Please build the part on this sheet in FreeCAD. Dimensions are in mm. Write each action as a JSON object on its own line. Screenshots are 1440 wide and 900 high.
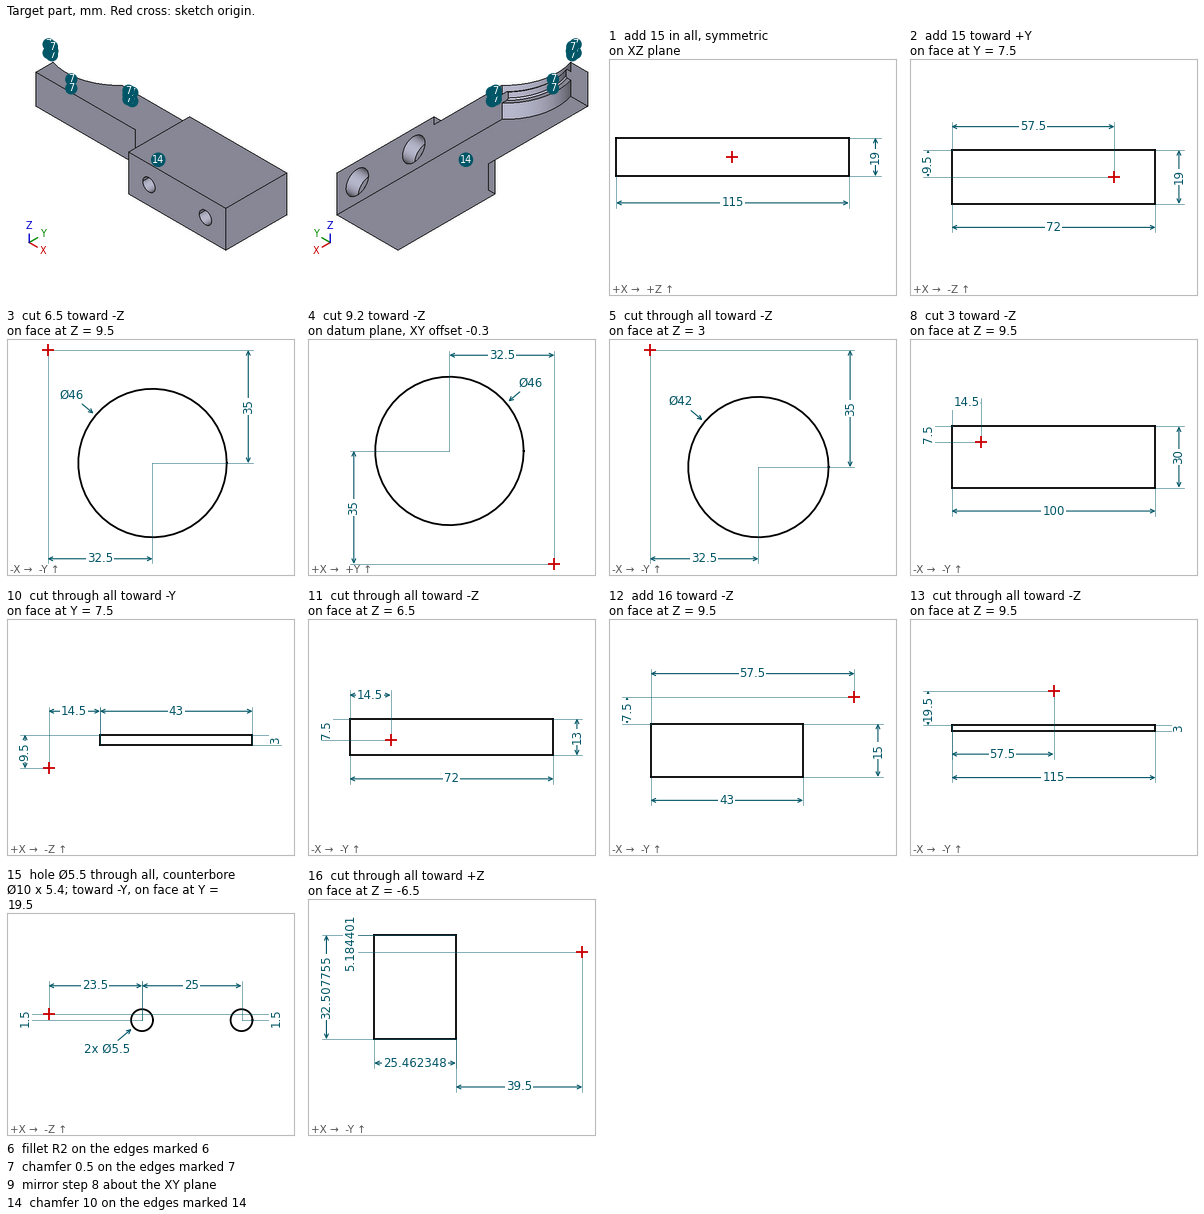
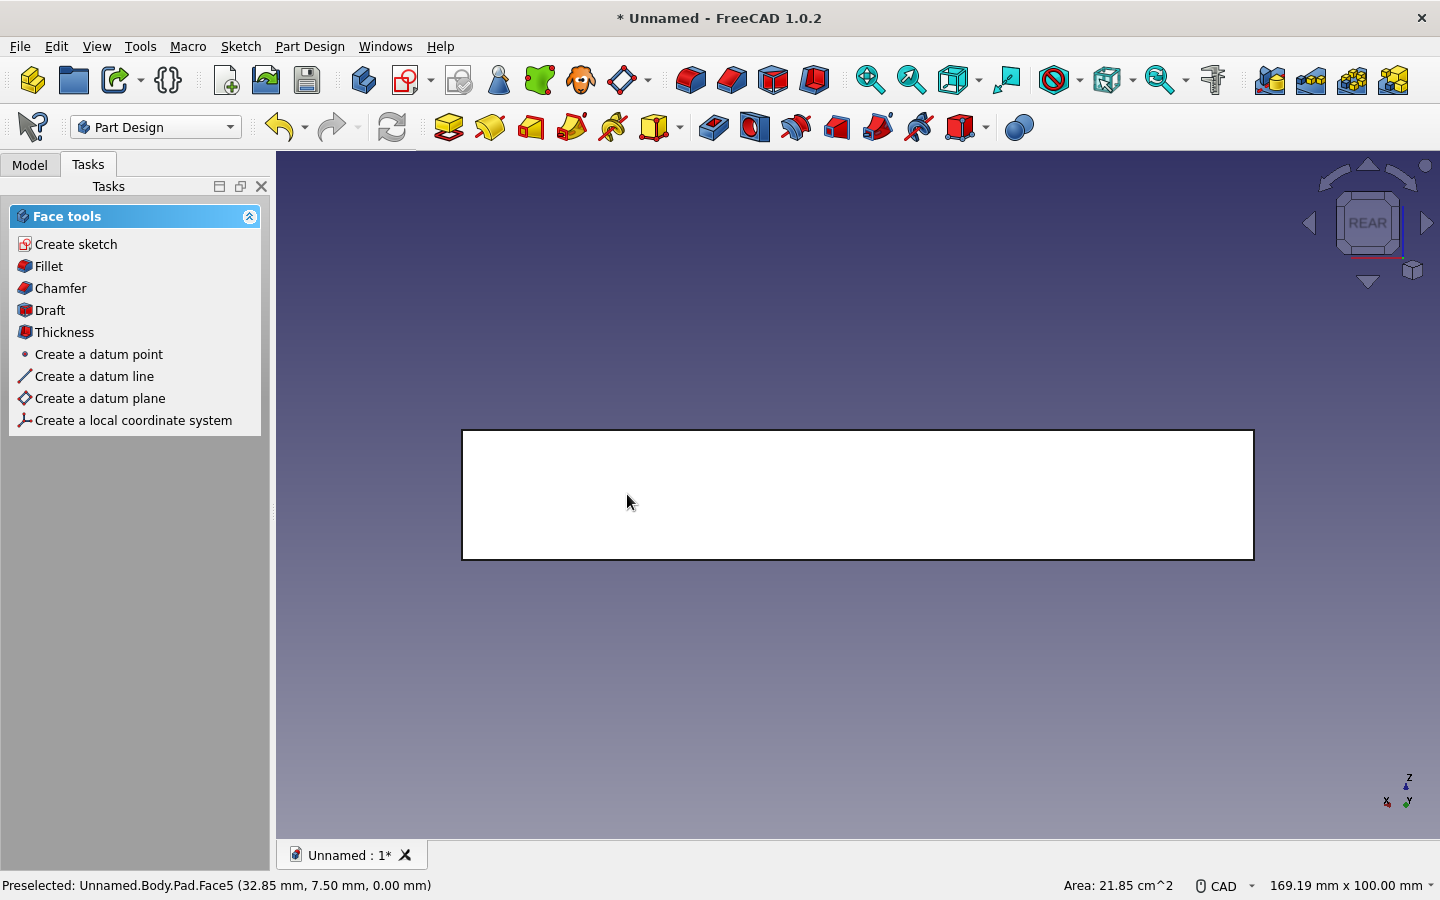
{"action": "left_click", "coordinate": [404, 80]}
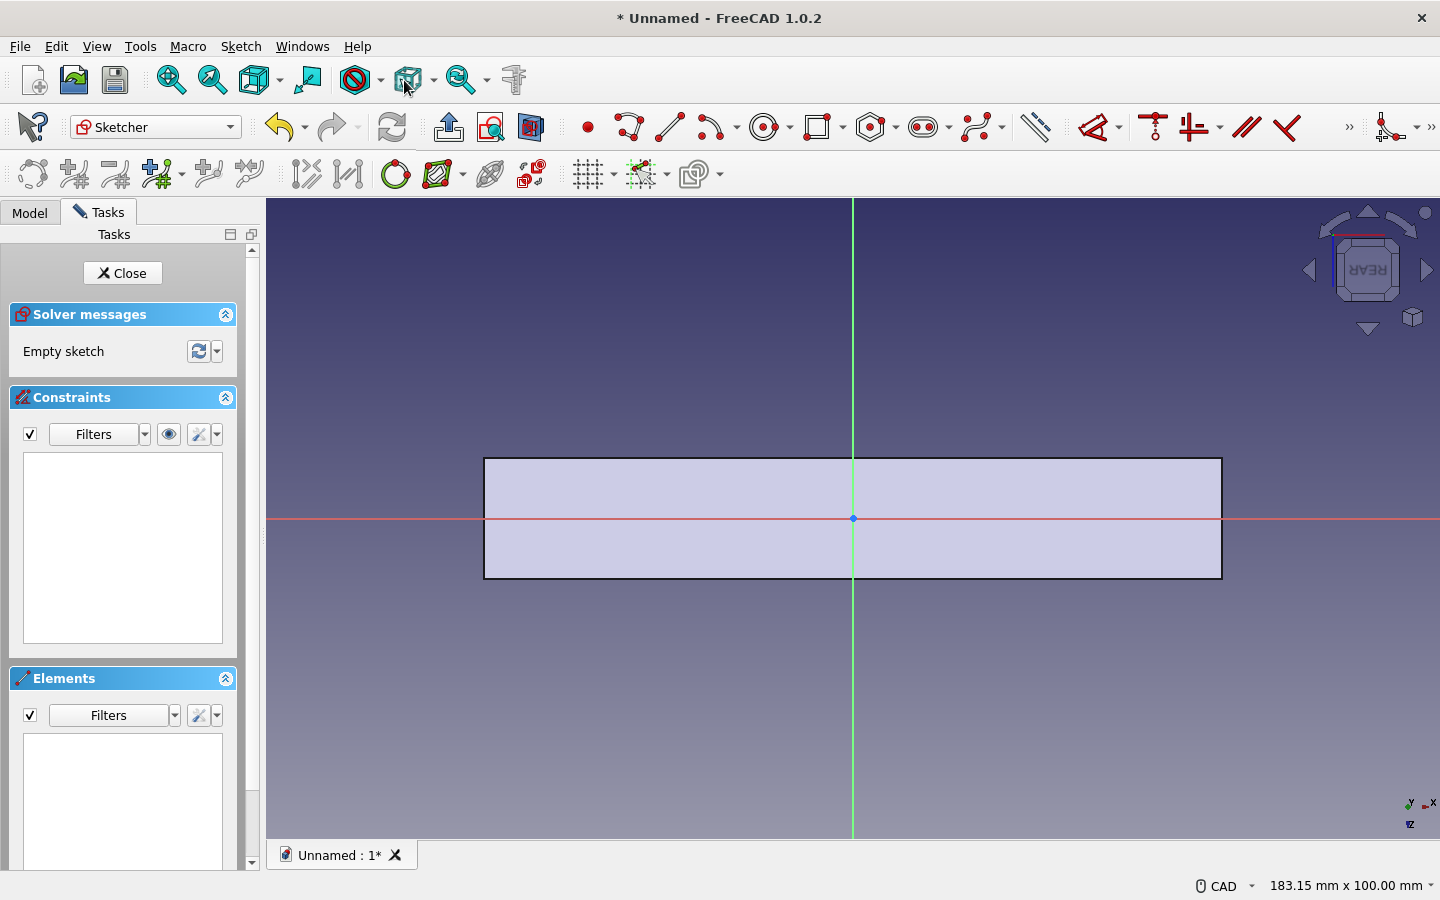
{"action": "scroll", "coordinate": [574, 519], "scroll_direction": "up", "scroll_amount": 2}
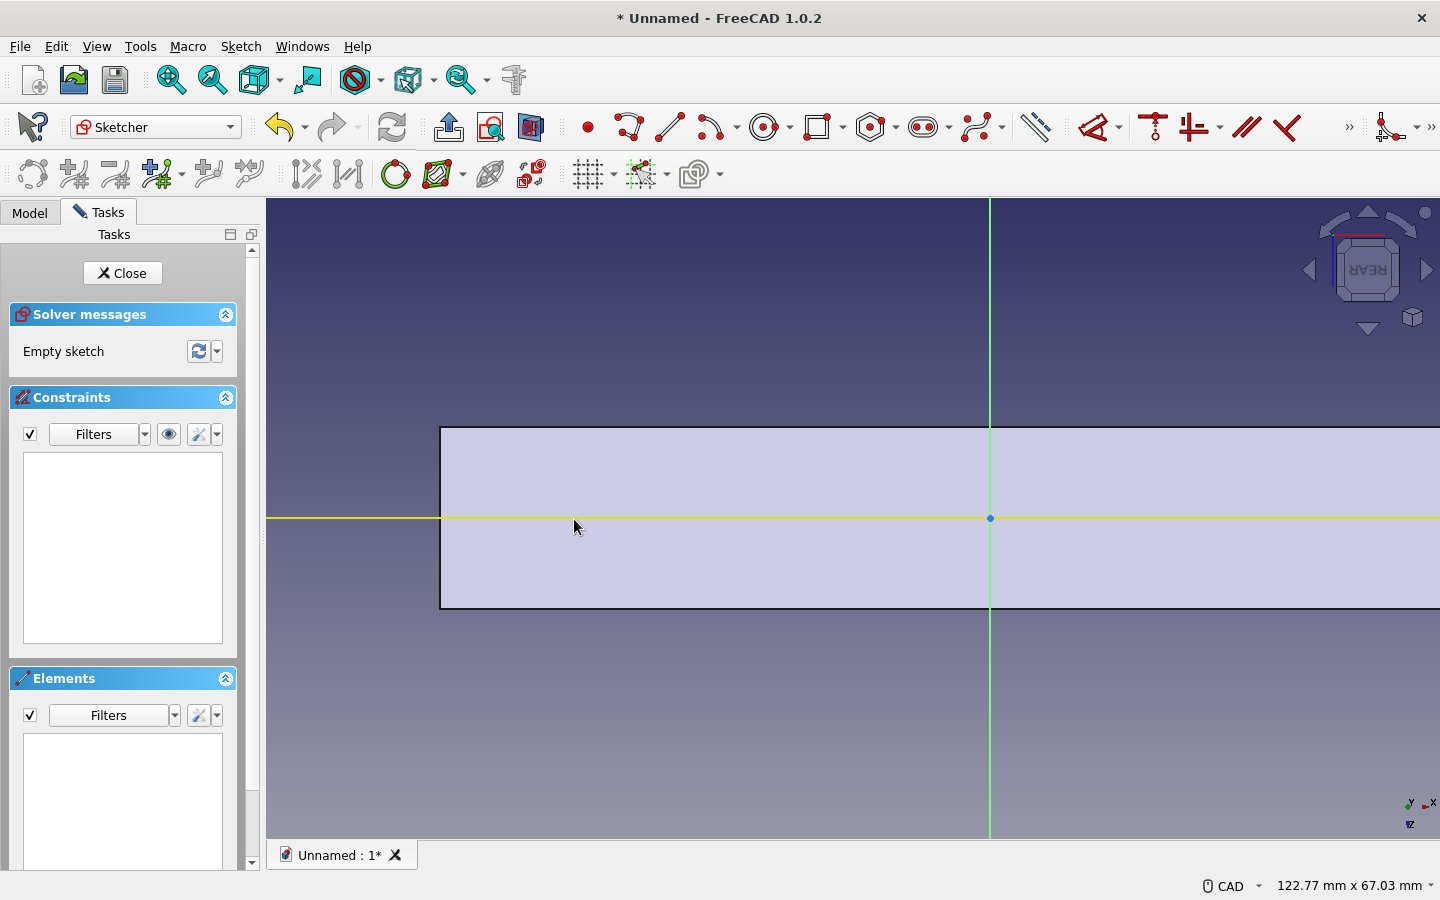
{"action": "left_click", "coordinate": [816, 128]}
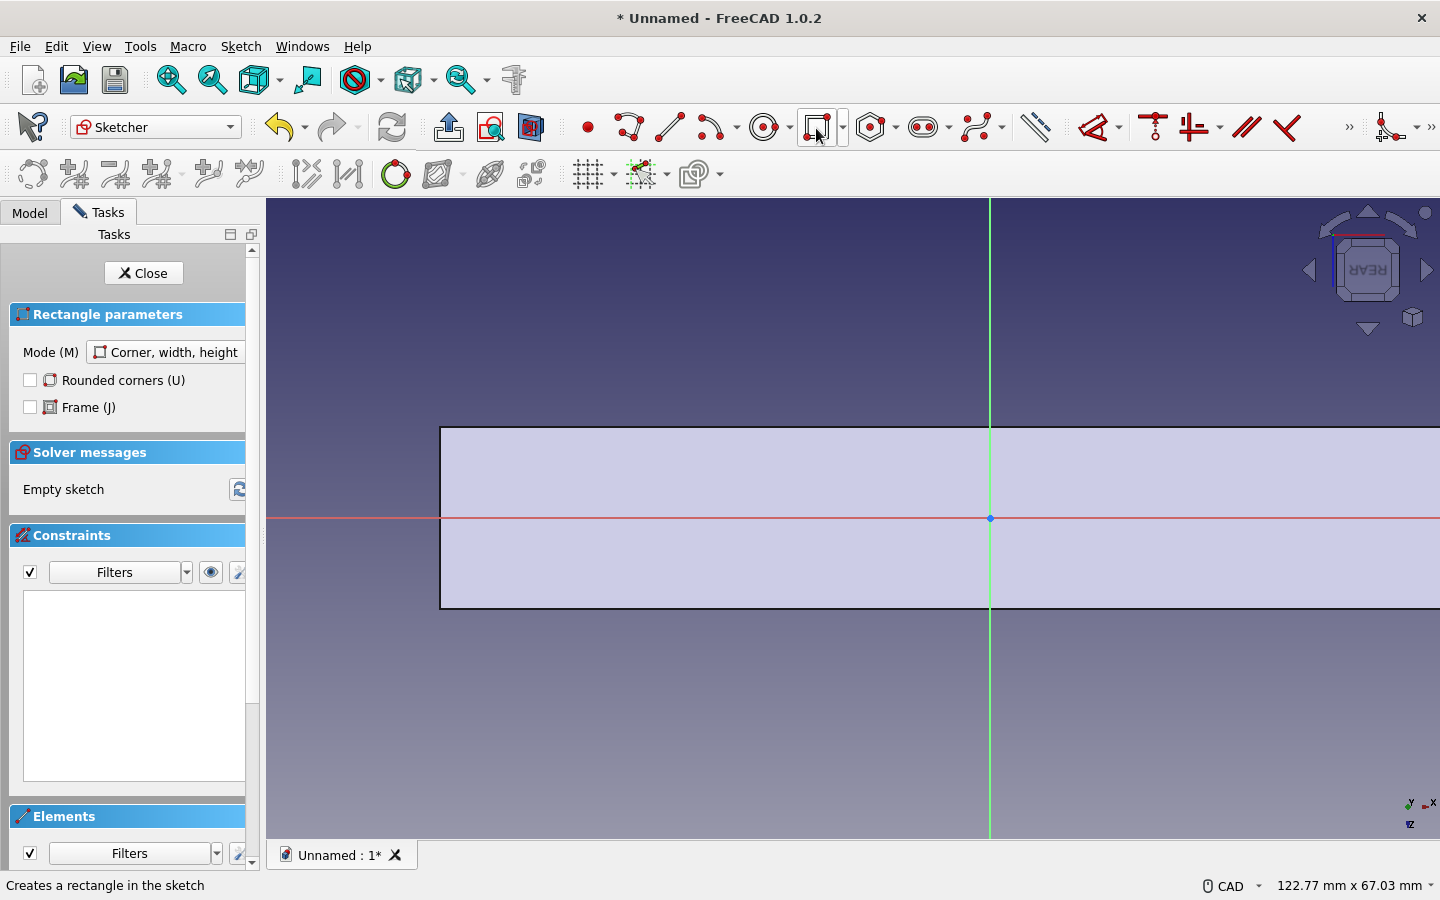
{"action": "left_click", "coordinate": [440, 427]}
{"action": "mouse_move", "coordinate": [1129, 609]}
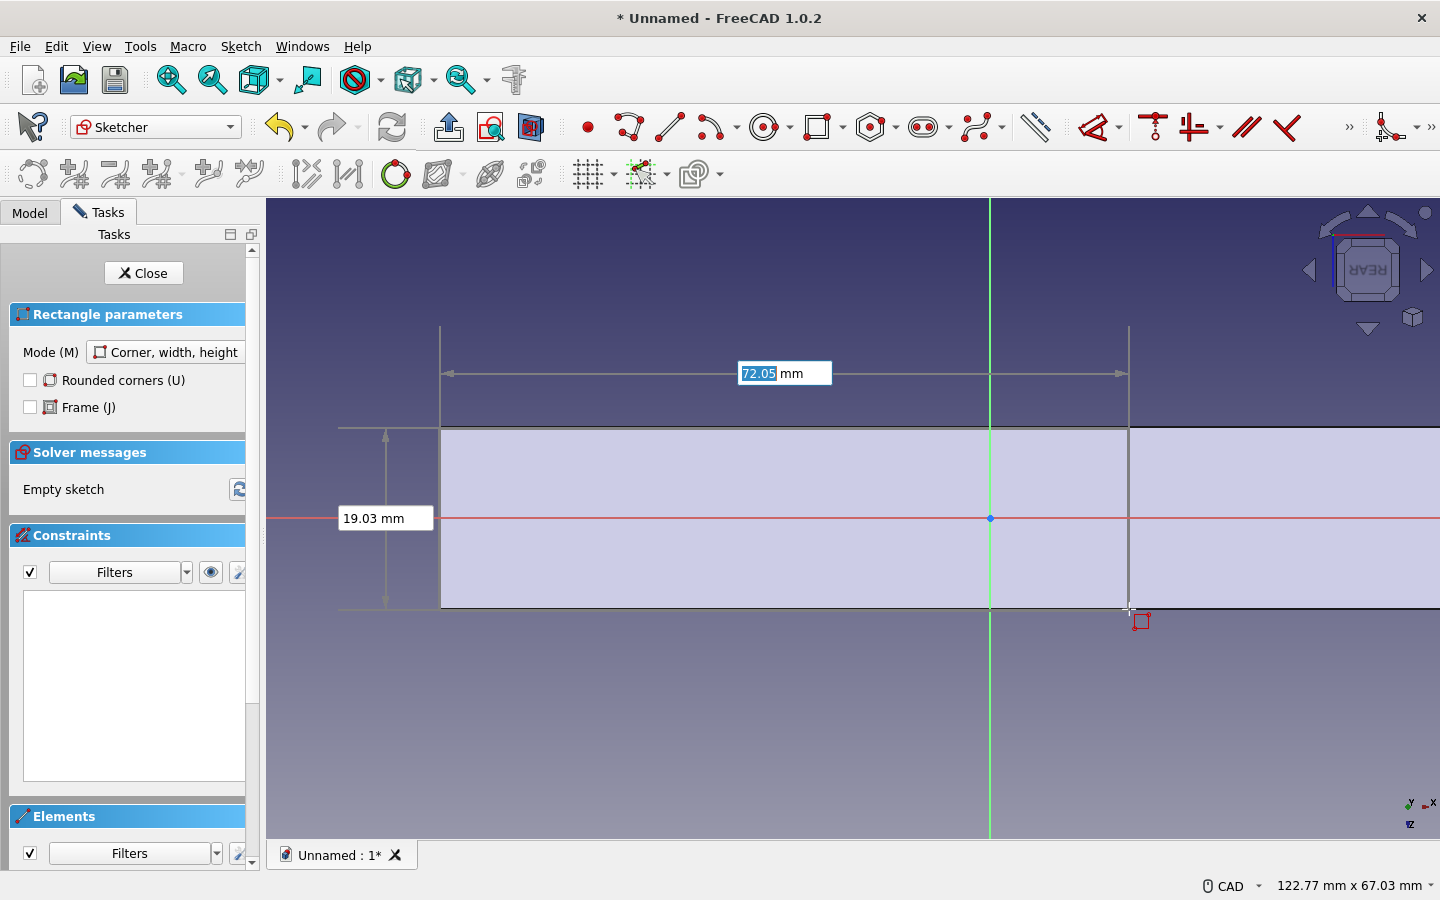
{"action": "type", "text": "72"}
{"action": "key", "text": "Tab"}
{"action": "type", "text": "19"}
{"action": "key", "text": "Return"}
{"action": "key", "text": "Escape"}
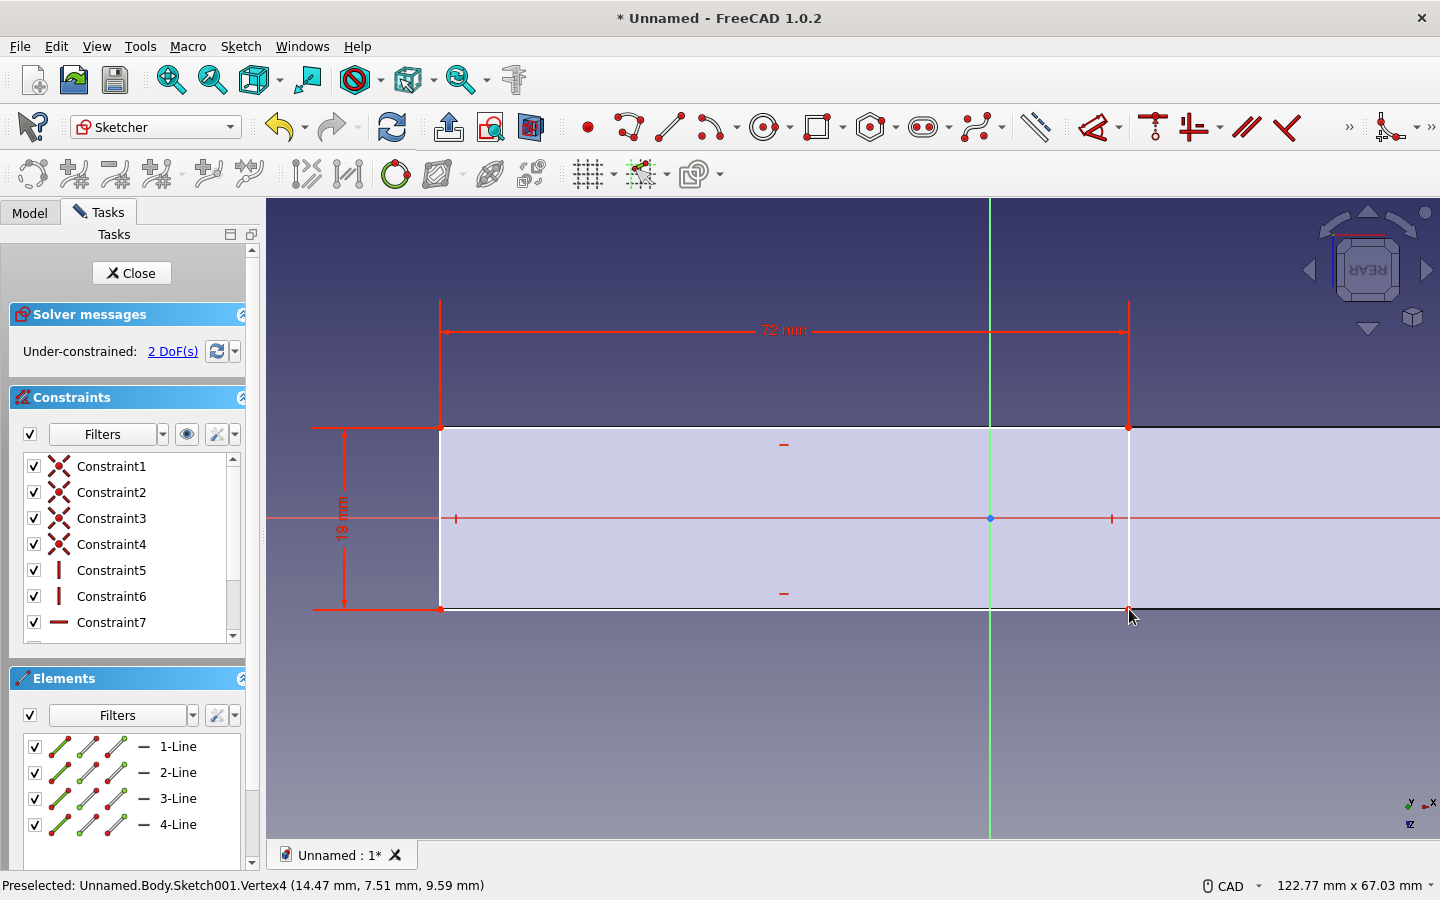
{"action": "left_click", "coordinate": [440, 428]}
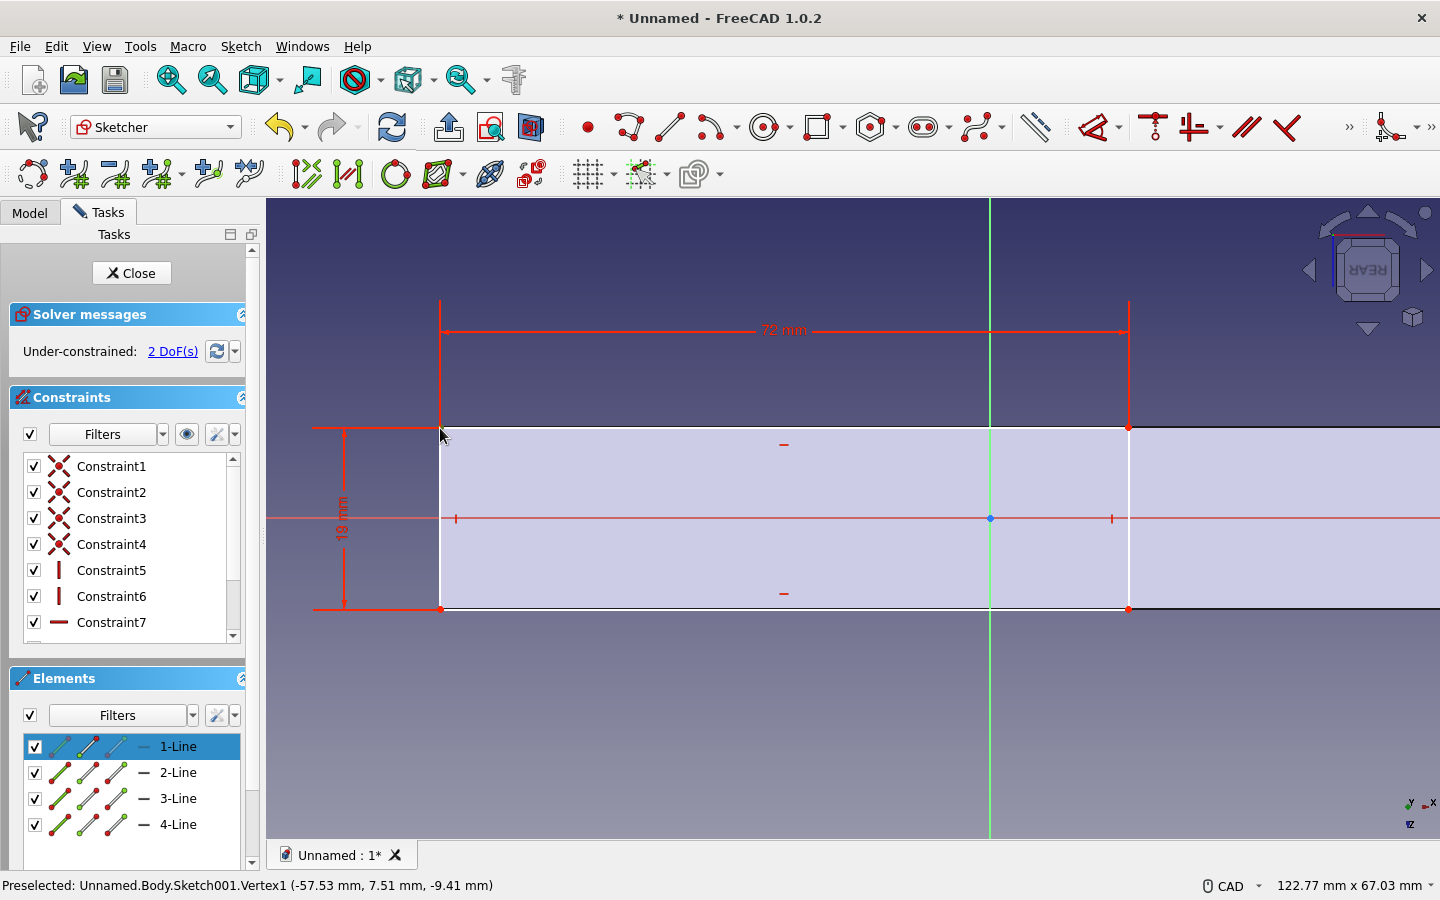
{"action": "left_click", "coordinate": [1118, 128]}